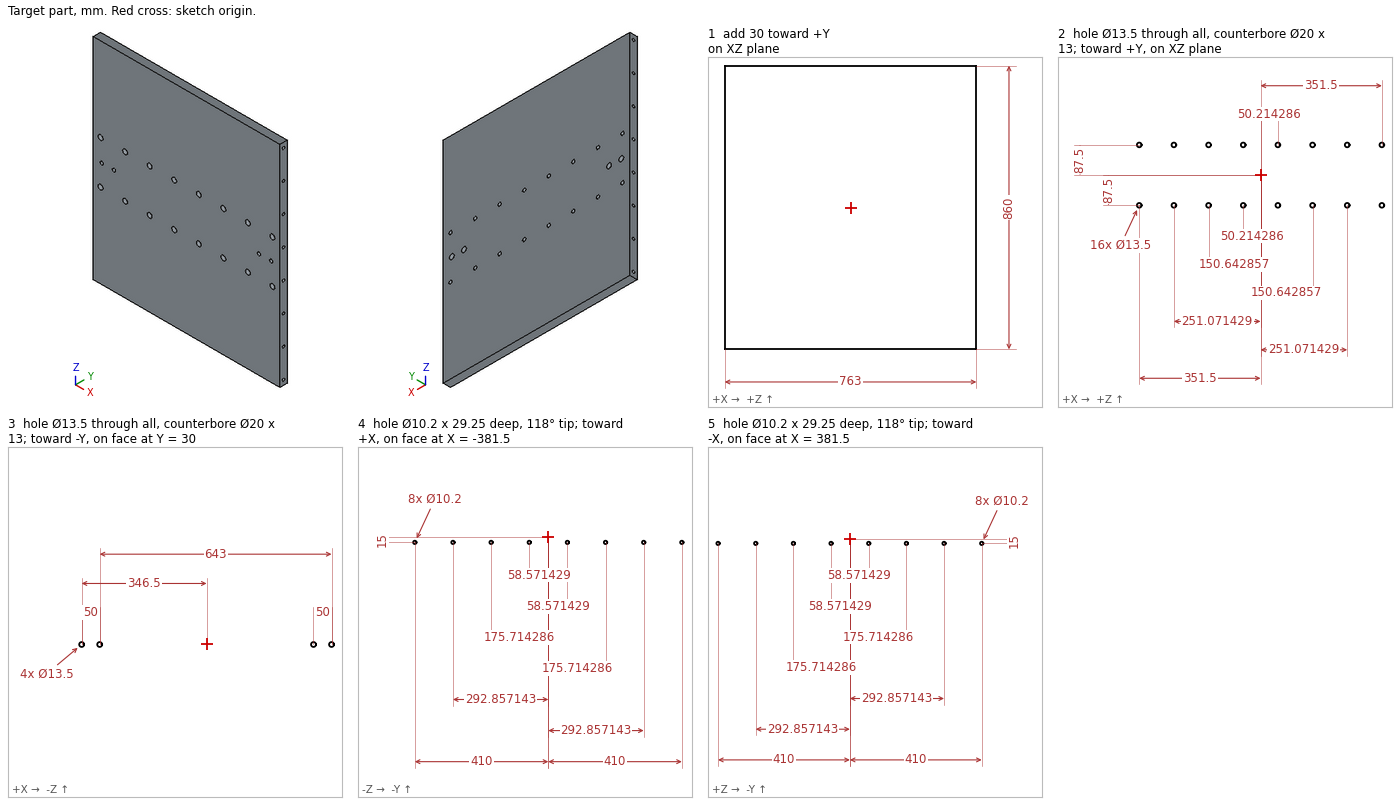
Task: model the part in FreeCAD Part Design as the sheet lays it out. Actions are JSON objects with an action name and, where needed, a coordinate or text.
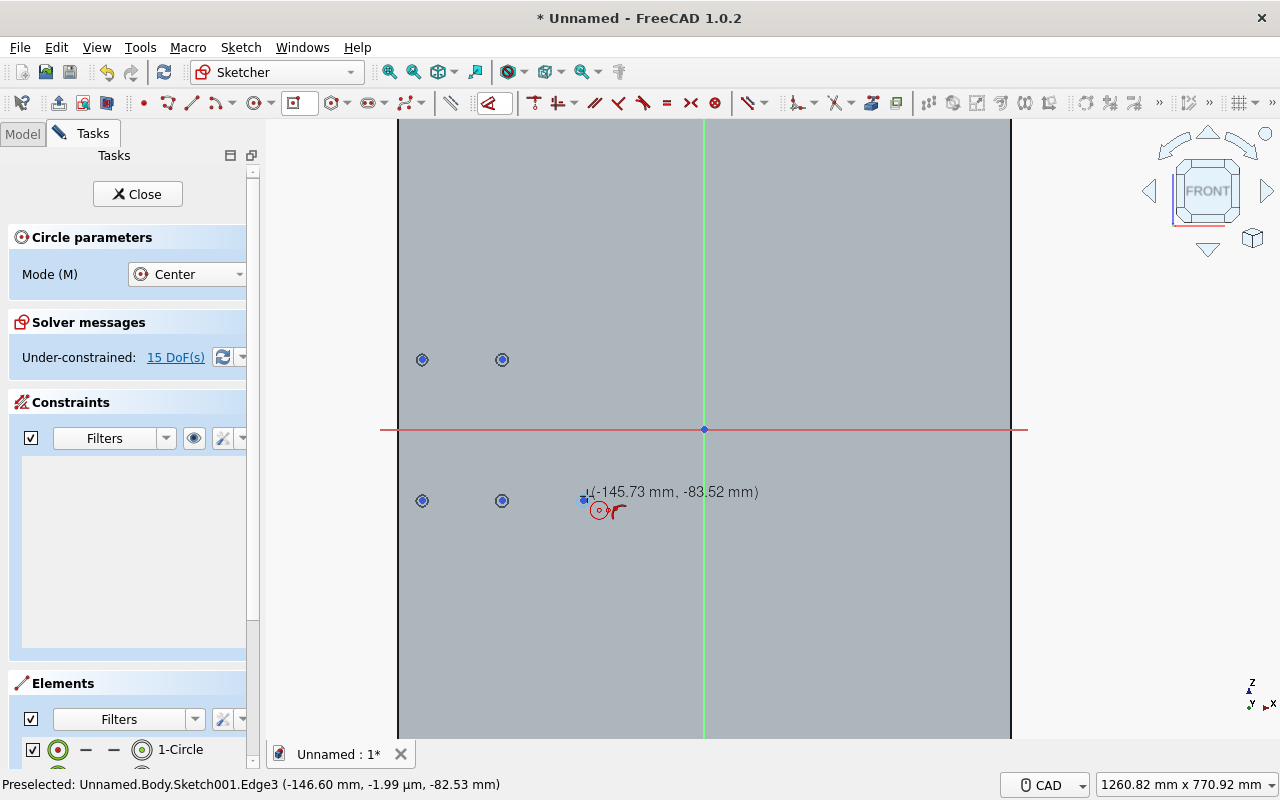
{"action": "scroll", "coordinate": [583, 359], "scroll_direction": "up", "scroll_amount": 8}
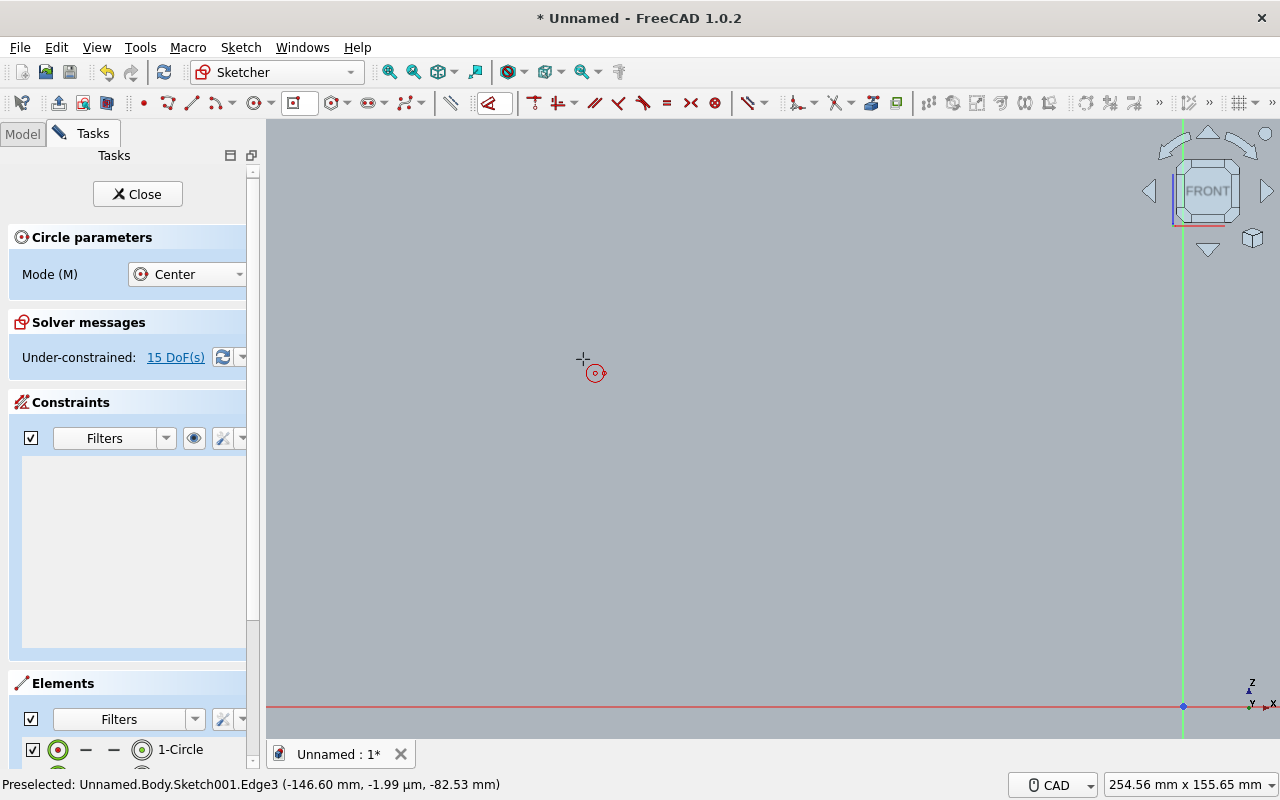
{"action": "scroll", "coordinate": [583, 359], "scroll_direction": "down", "scroll_amount": 8}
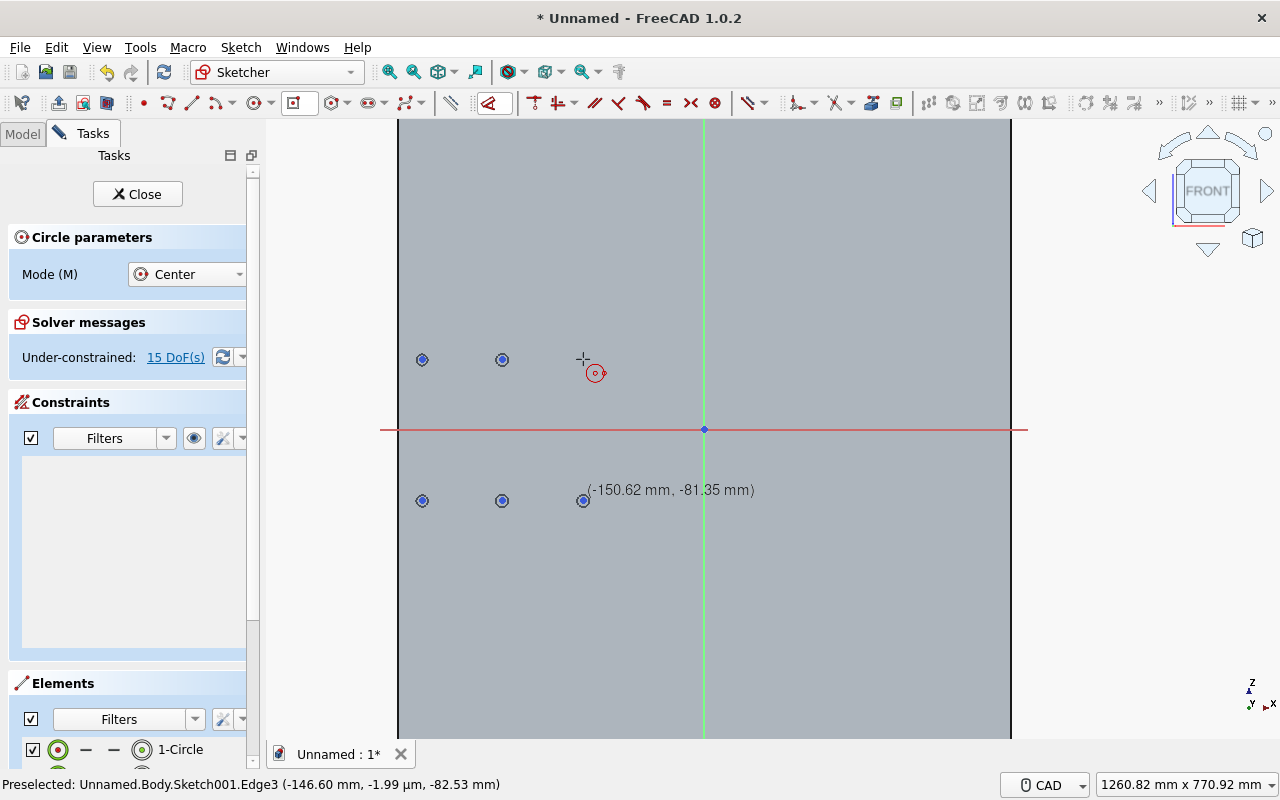
{"action": "left_click", "coordinate": [583, 359]}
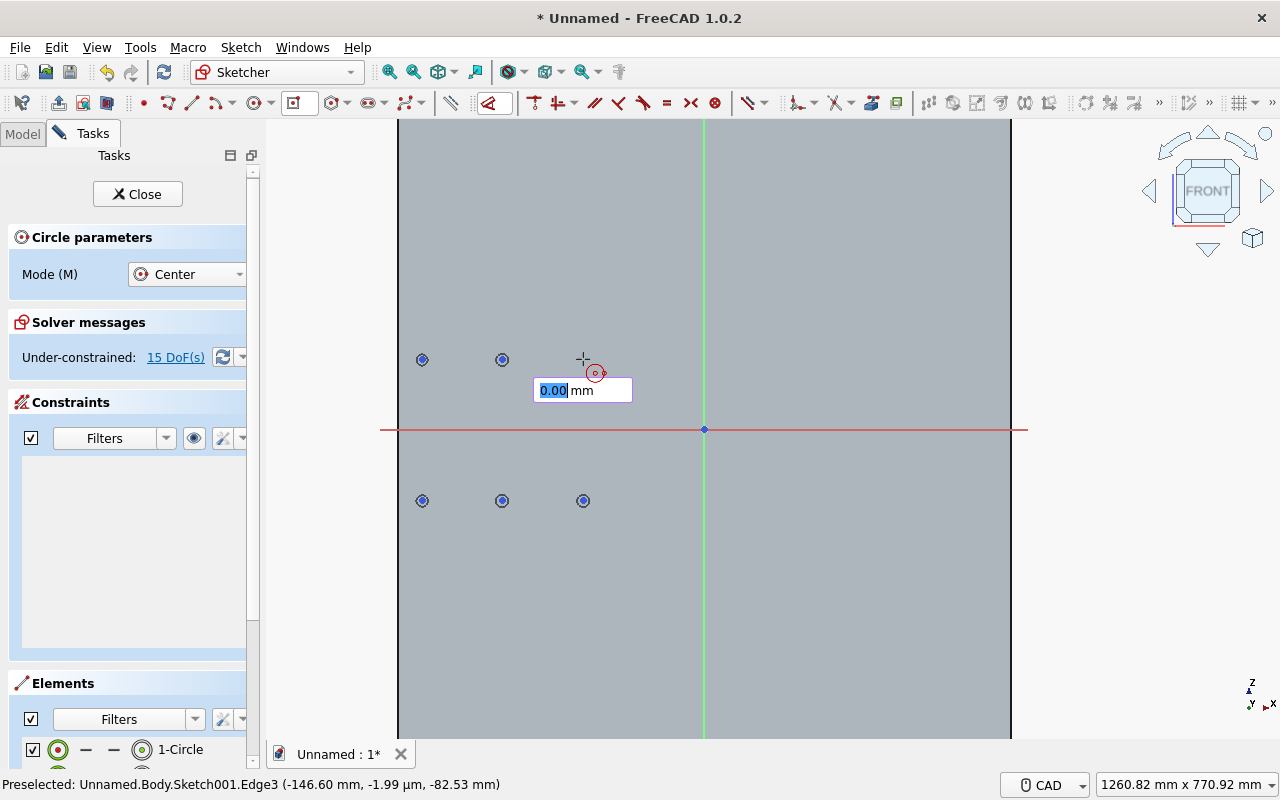
{"action": "scroll", "coordinate": [587, 355], "scroll_direction": "up", "scroll_amount": 6}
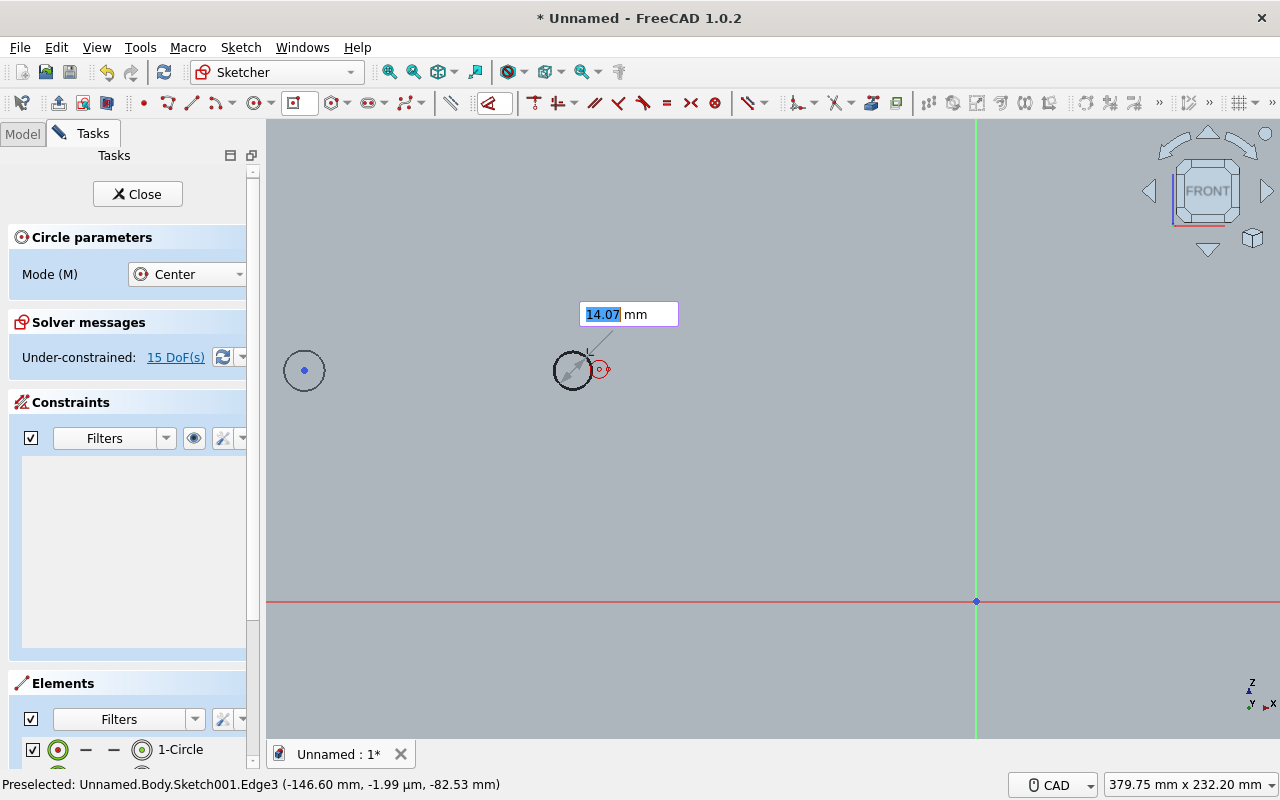
{"action": "left_click", "coordinate": [587, 355]}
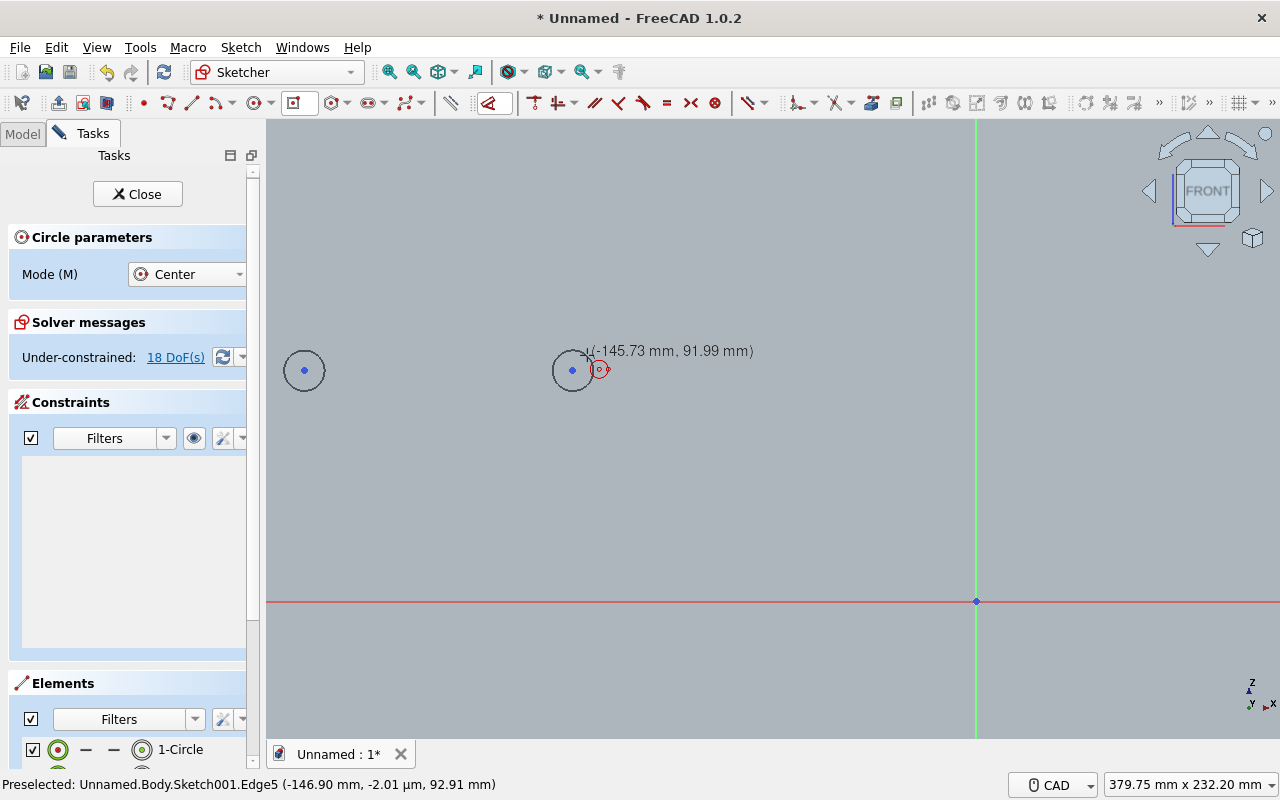
{"action": "scroll", "coordinate": [587, 355], "scroll_direction": "down", "scroll_amount": 6}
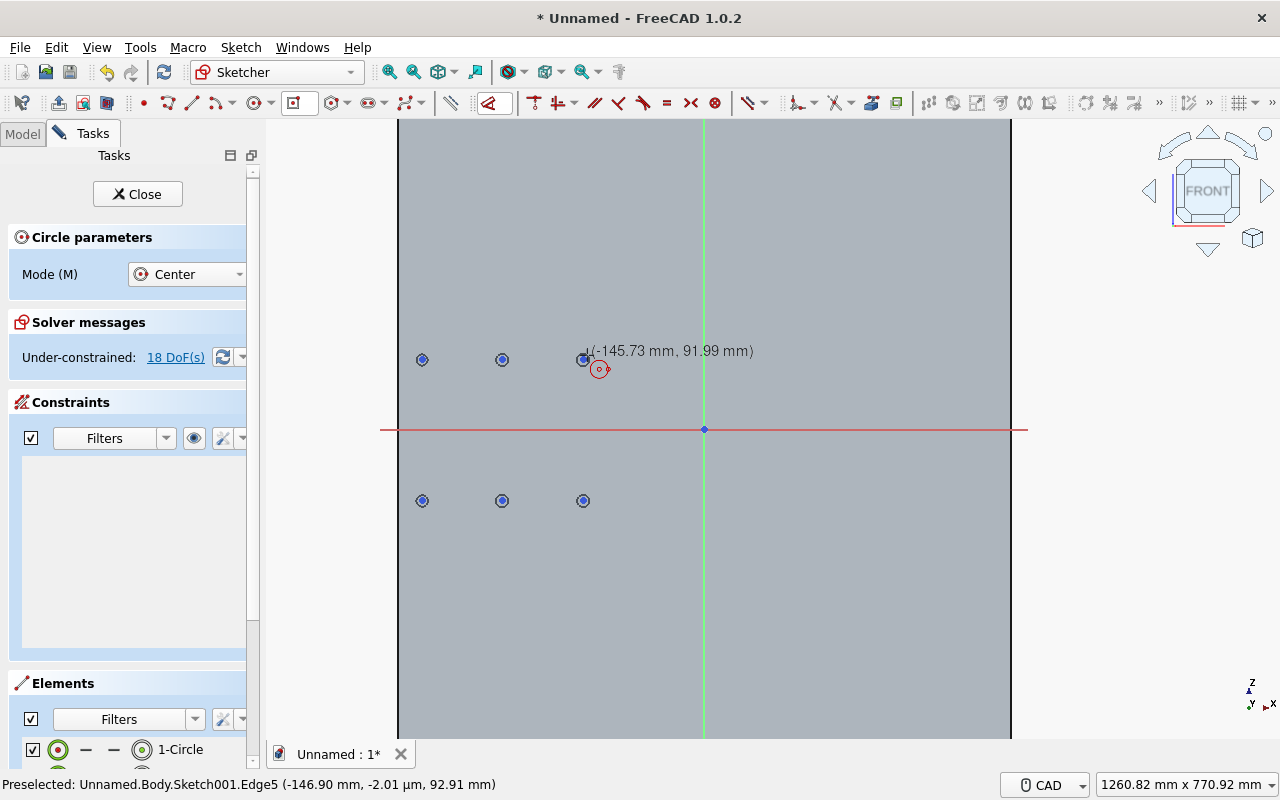
{"action": "scroll", "coordinate": [664, 500], "scroll_direction": "up", "scroll_amount": 8}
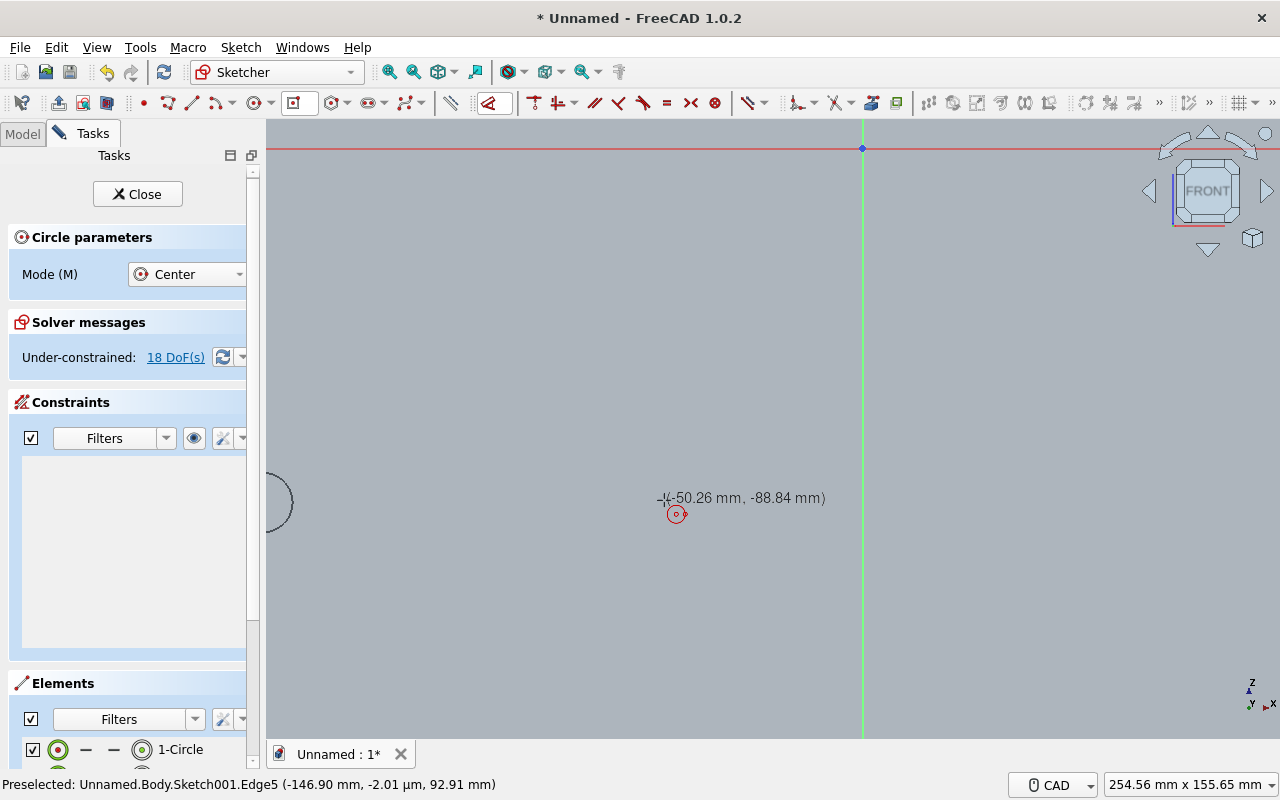
{"action": "scroll", "coordinate": [664, 500], "scroll_direction": "down", "scroll_amount": 8}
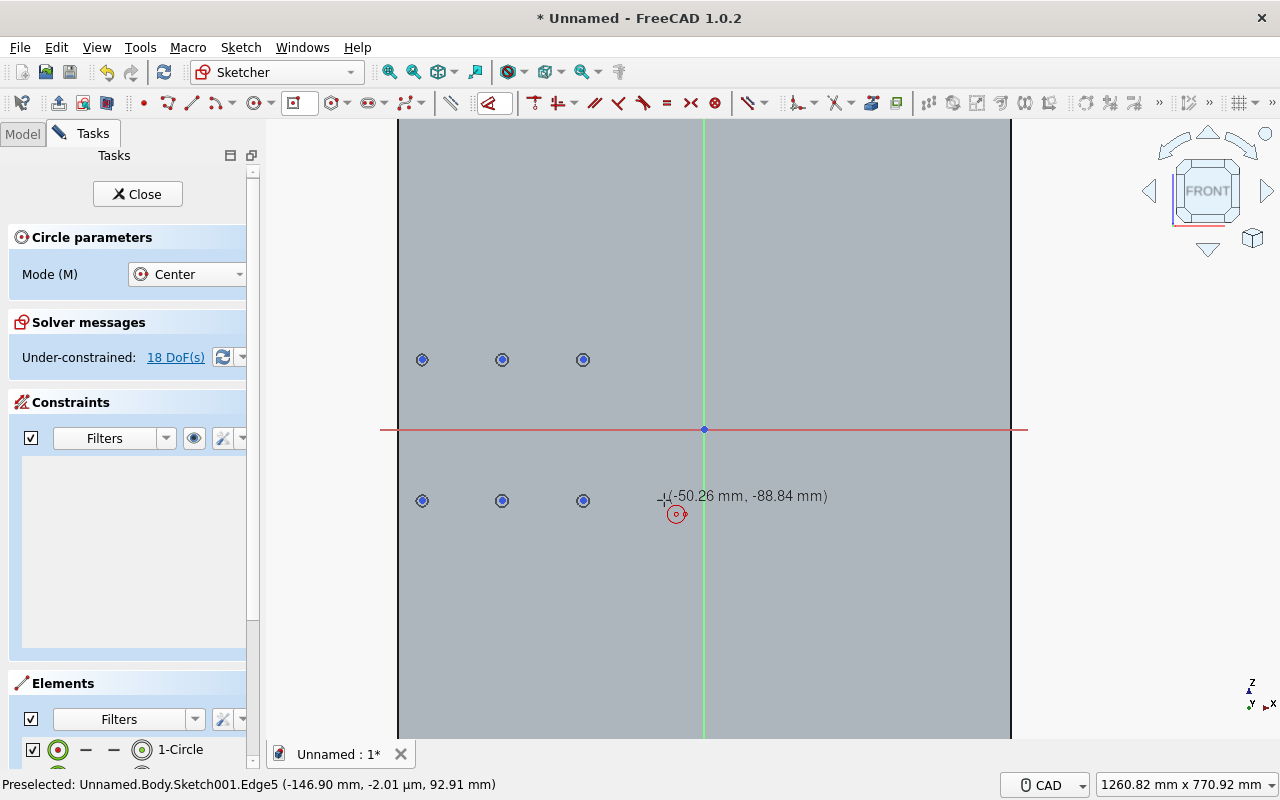
{"action": "left_click", "coordinate": [664, 500]}